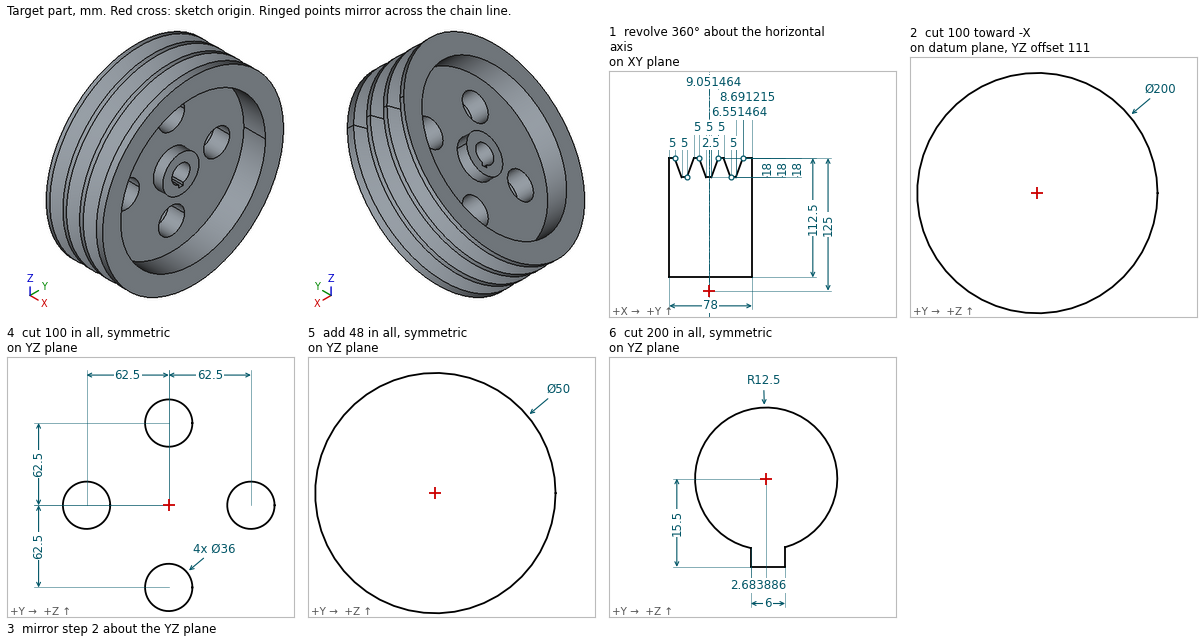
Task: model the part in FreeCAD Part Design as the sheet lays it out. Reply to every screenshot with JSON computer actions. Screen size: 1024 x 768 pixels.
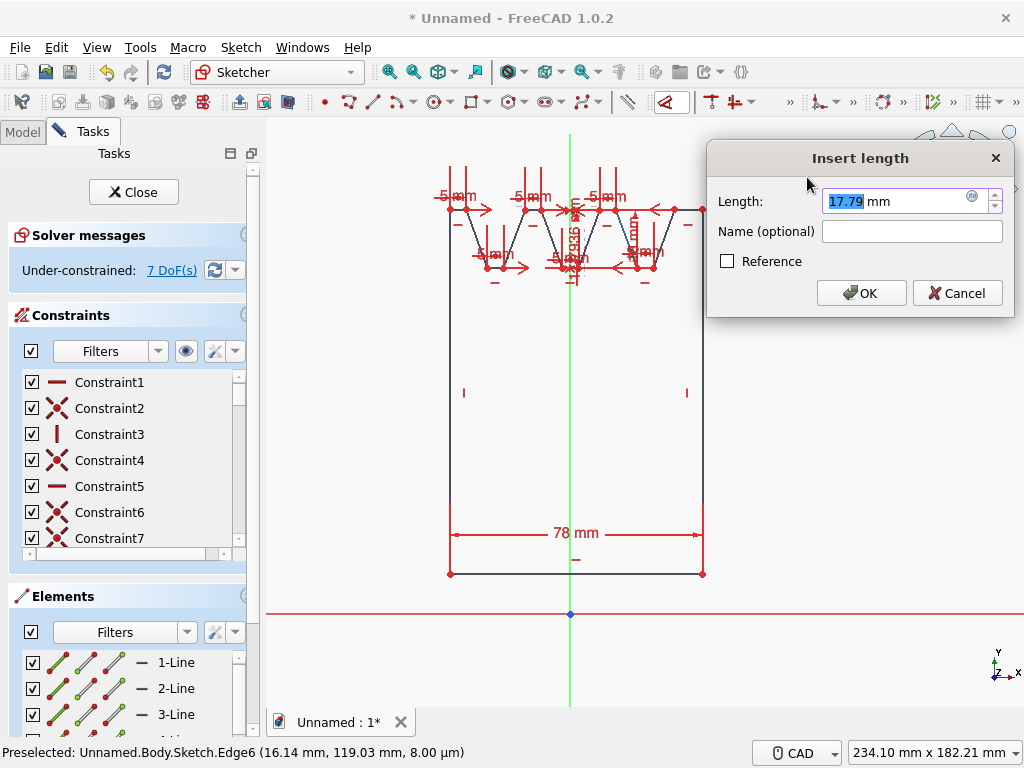
{"action": "type", "text": "18"}
{"action": "key", "text": "Return"}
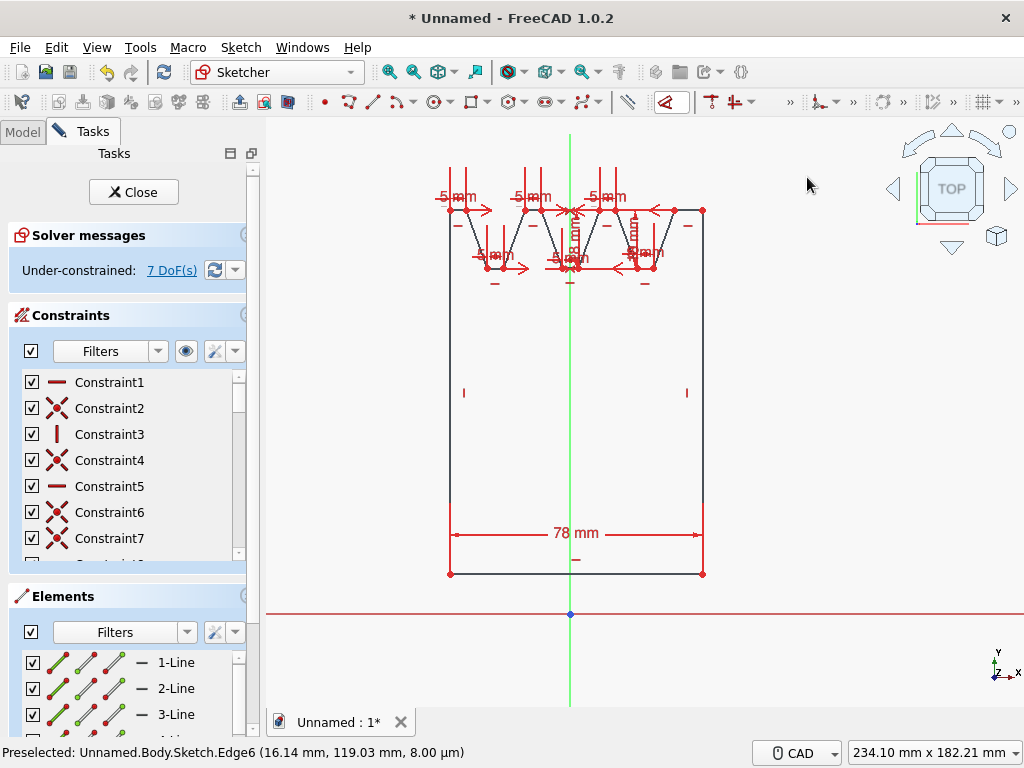
{"action": "left_click", "coordinate": [593, 228]}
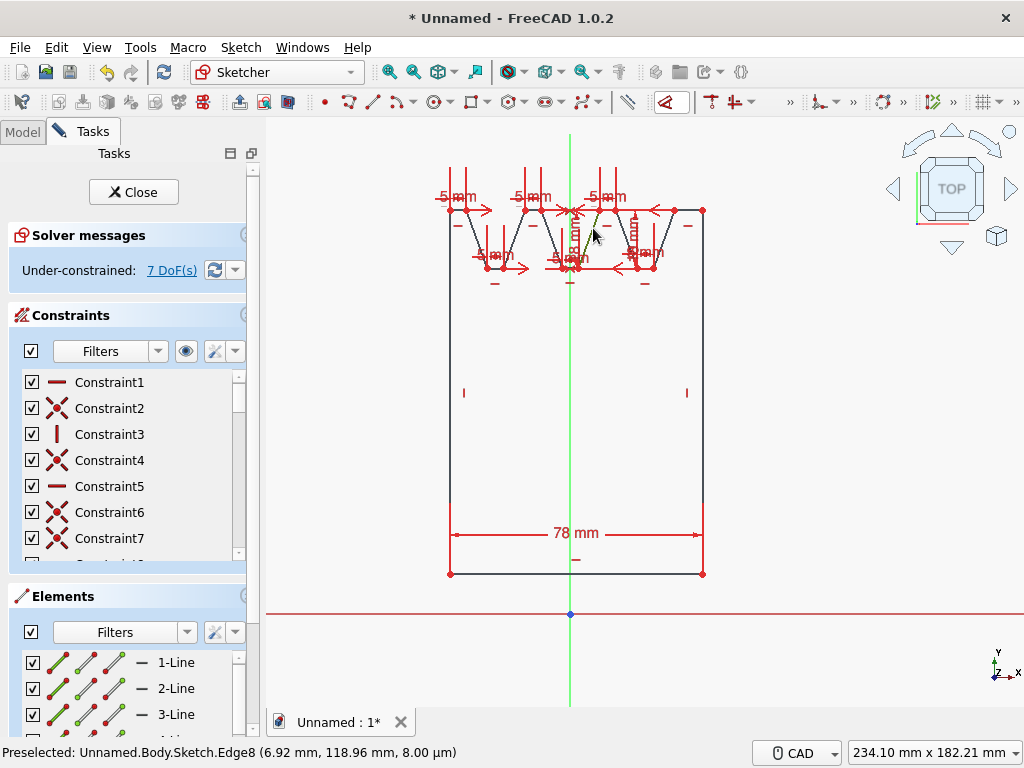
{"action": "left_click", "coordinate": [684, 102]}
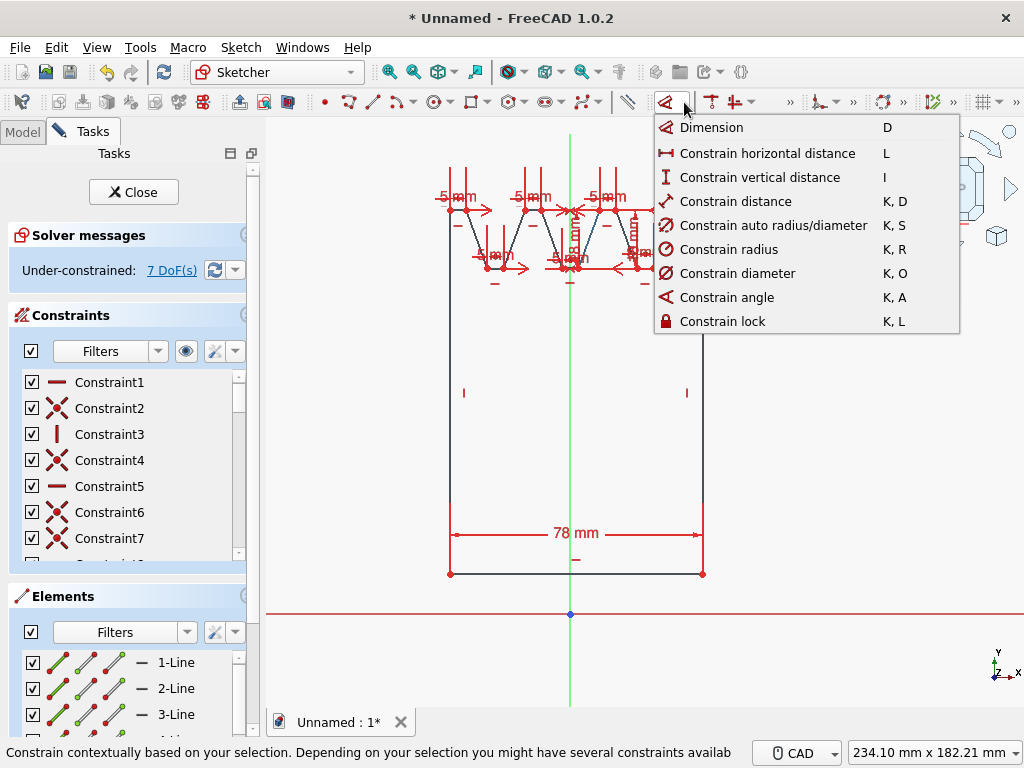
{"action": "left_click", "coordinate": [807, 177]}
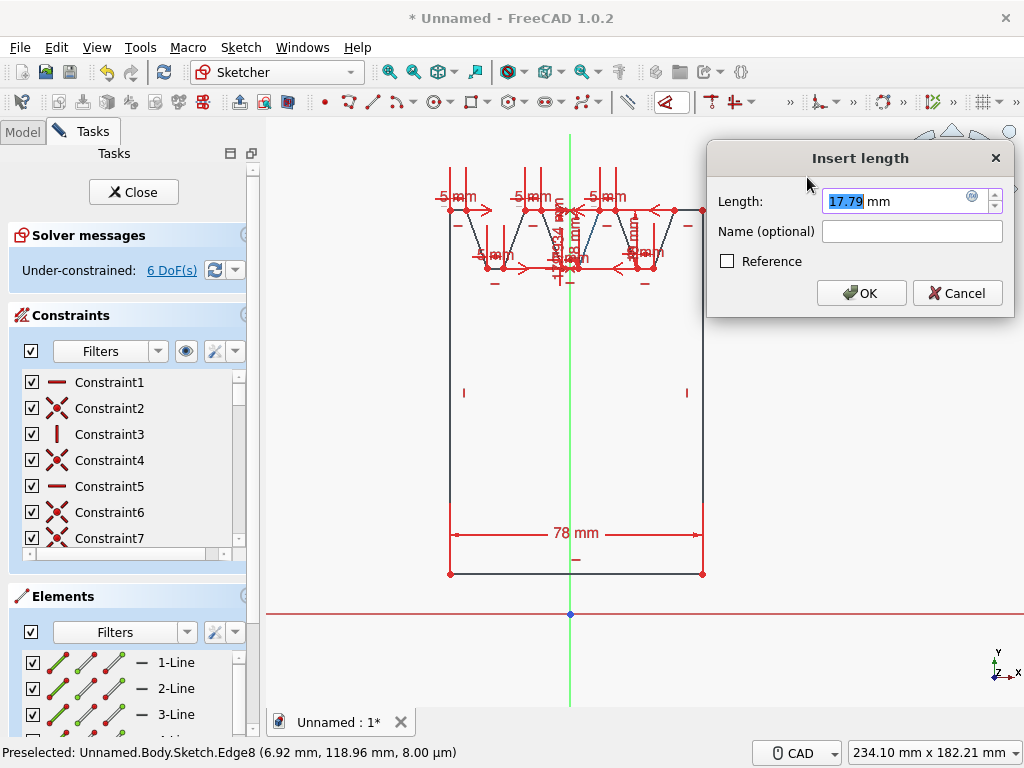
{"action": "type", "text": "18"}
{"action": "key", "text": "Return"}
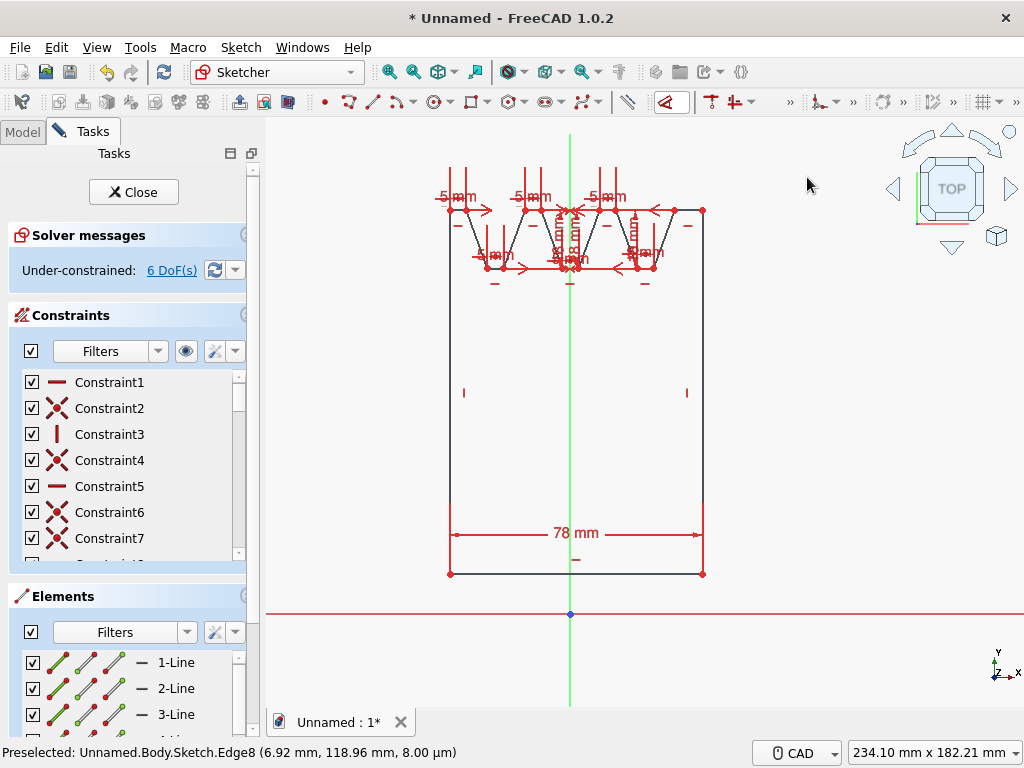
{"action": "left_click", "coordinate": [703, 210]}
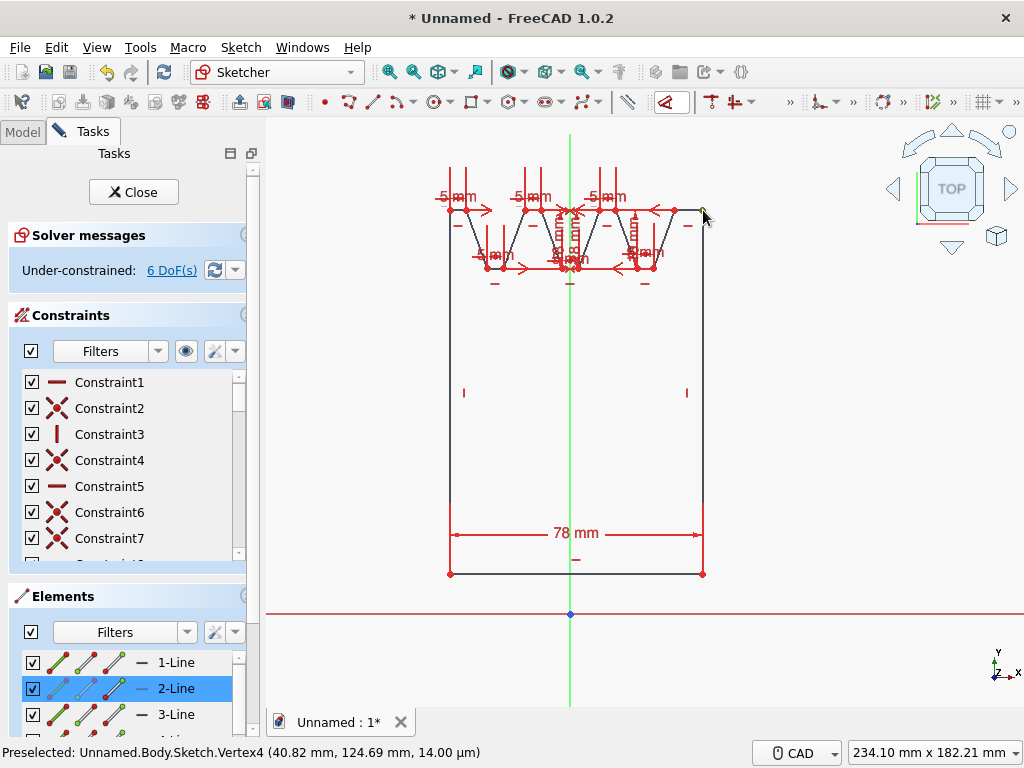
{"action": "left_click", "coordinate": [684, 102]}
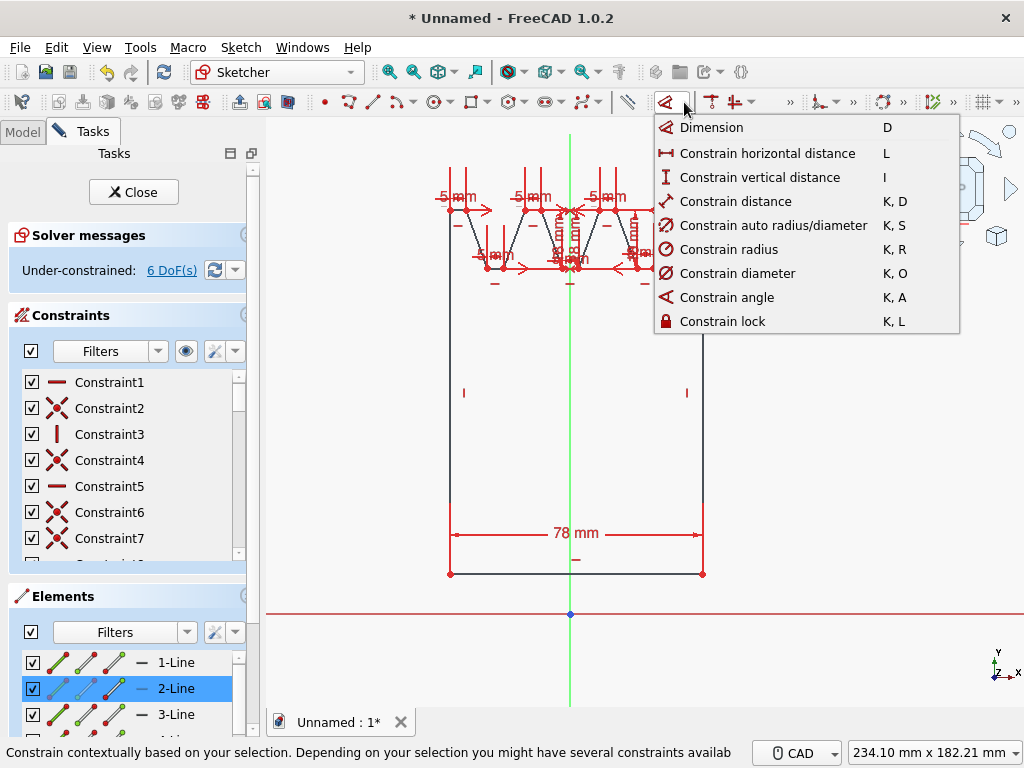
{"action": "left_click", "coordinate": [807, 177]}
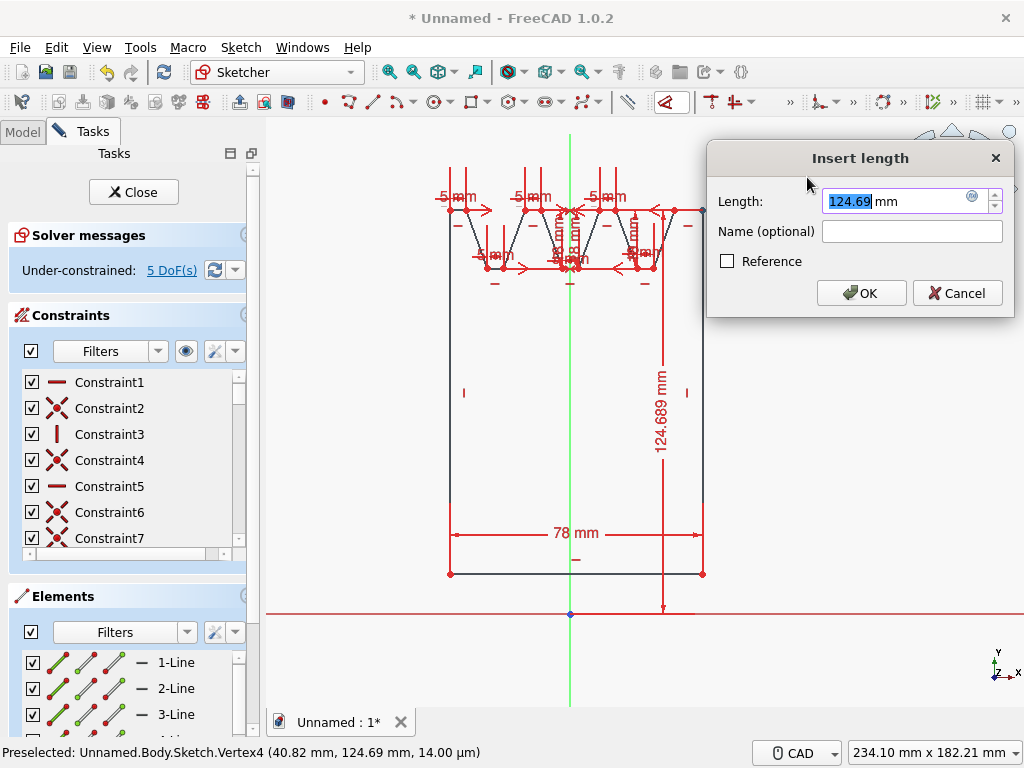
{"action": "type", "text": "125"}
{"action": "key", "text": "Return"}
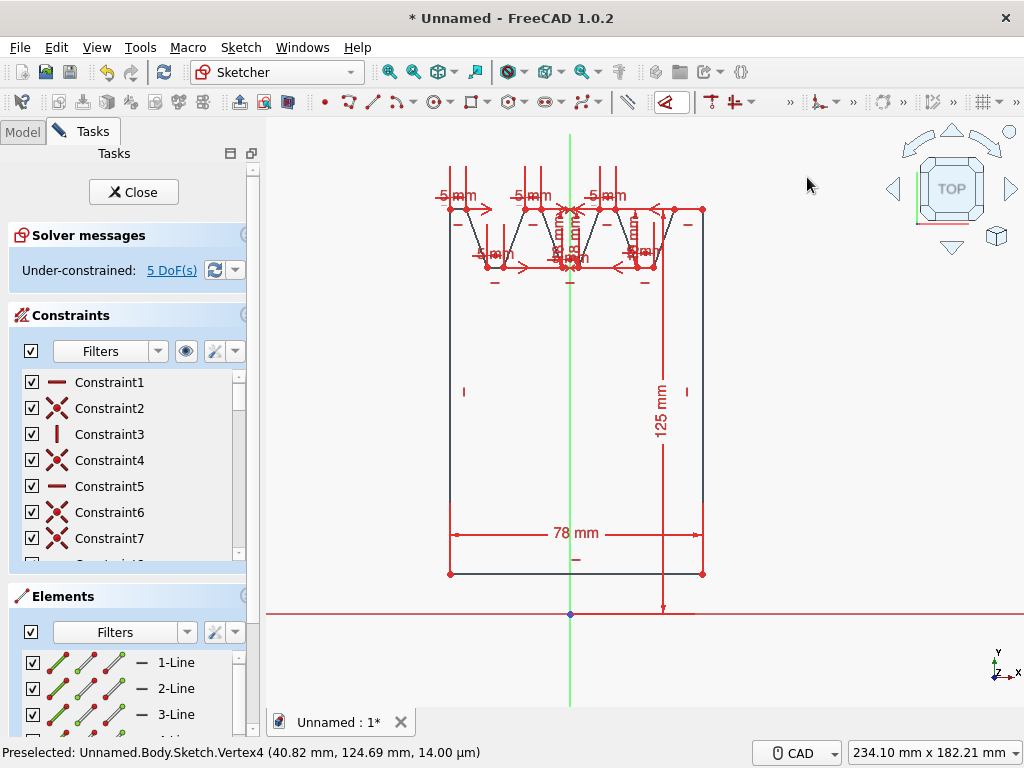
{"action": "scroll", "coordinate": [579, 268], "scroll_direction": "up", "scroll_amount": 8}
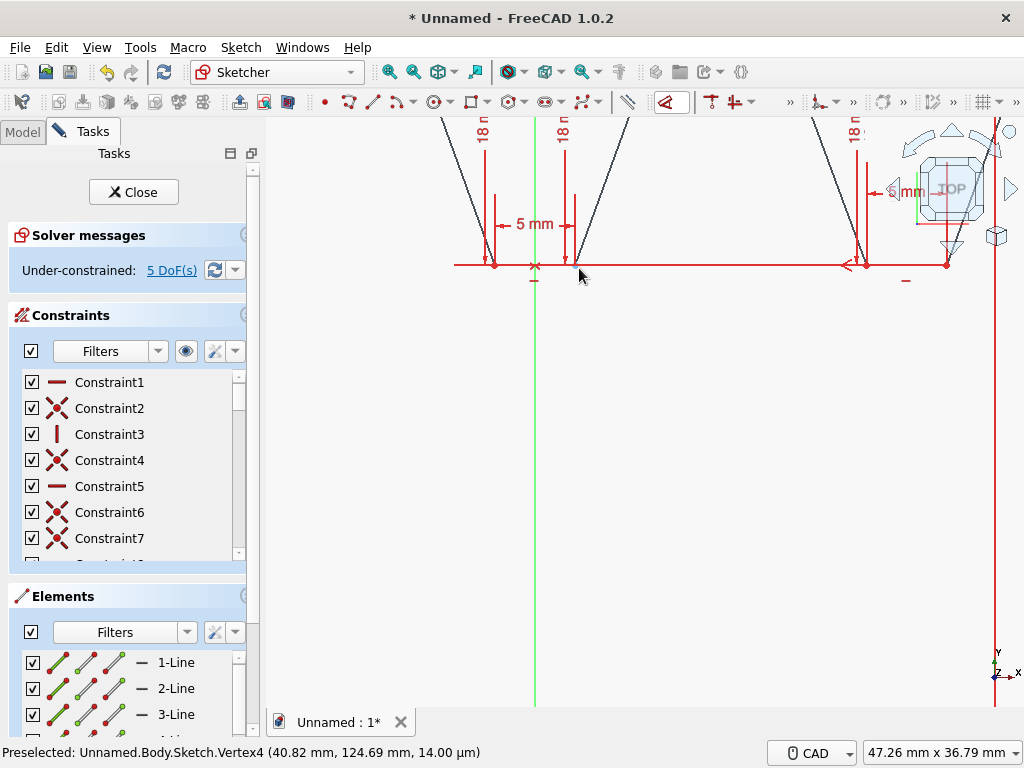
{"action": "left_click", "coordinate": [575, 265]}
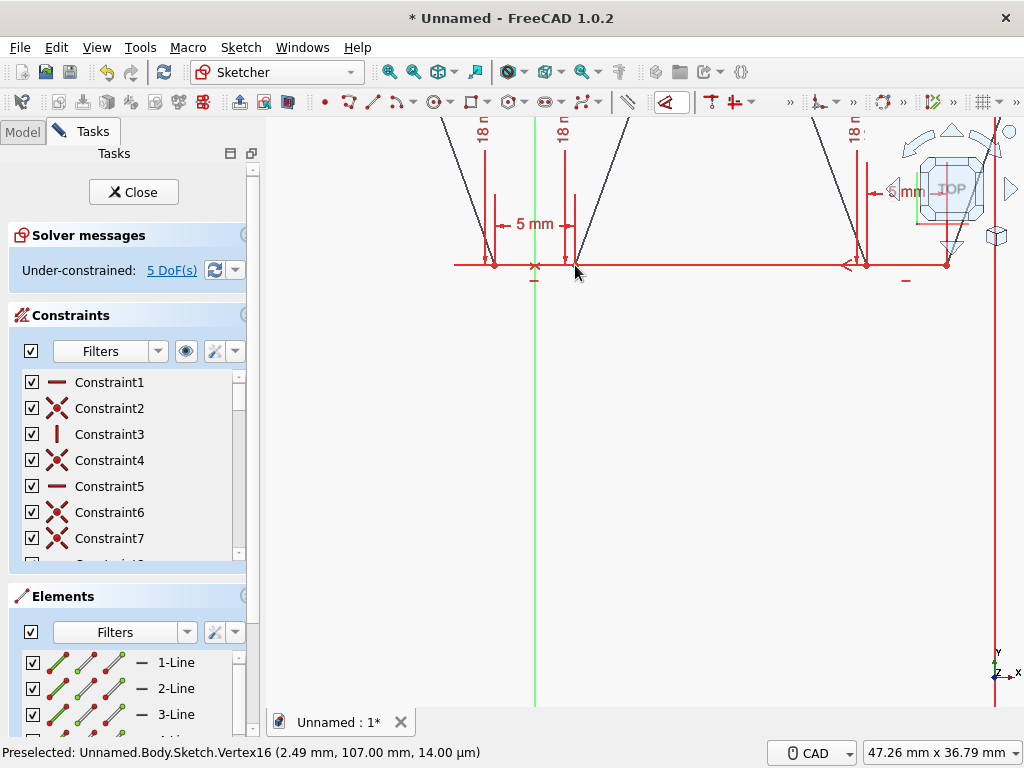
{"action": "key", "text": "l"}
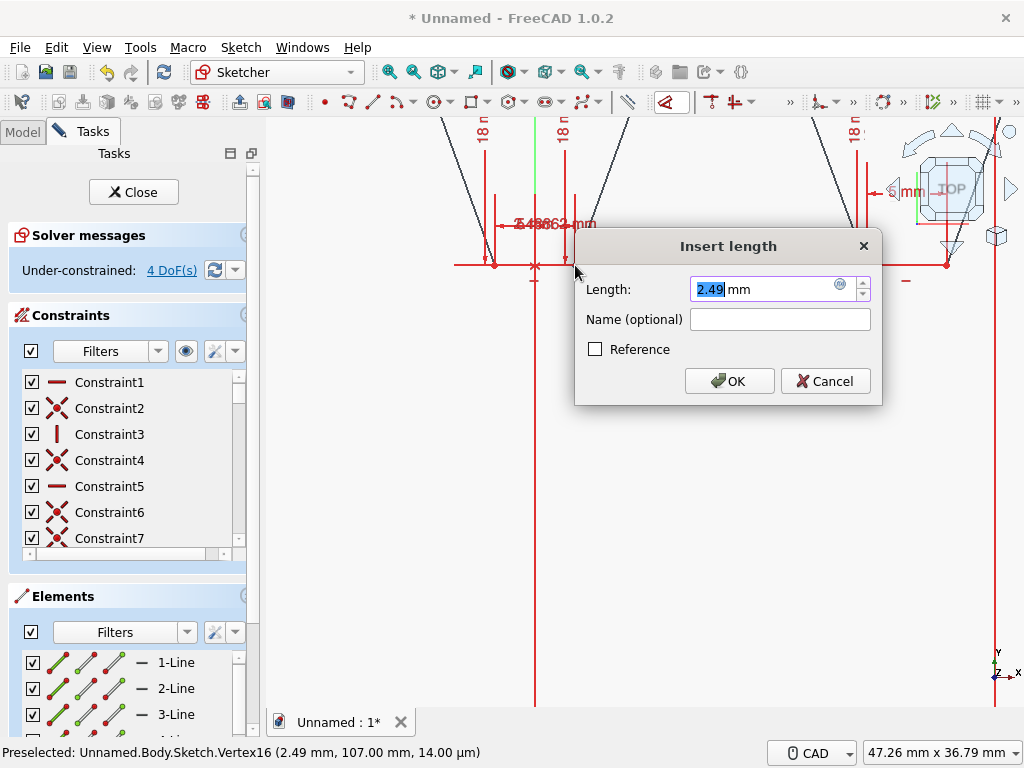
{"action": "type", "text": "2.5"}
{"action": "key", "text": "Return"}